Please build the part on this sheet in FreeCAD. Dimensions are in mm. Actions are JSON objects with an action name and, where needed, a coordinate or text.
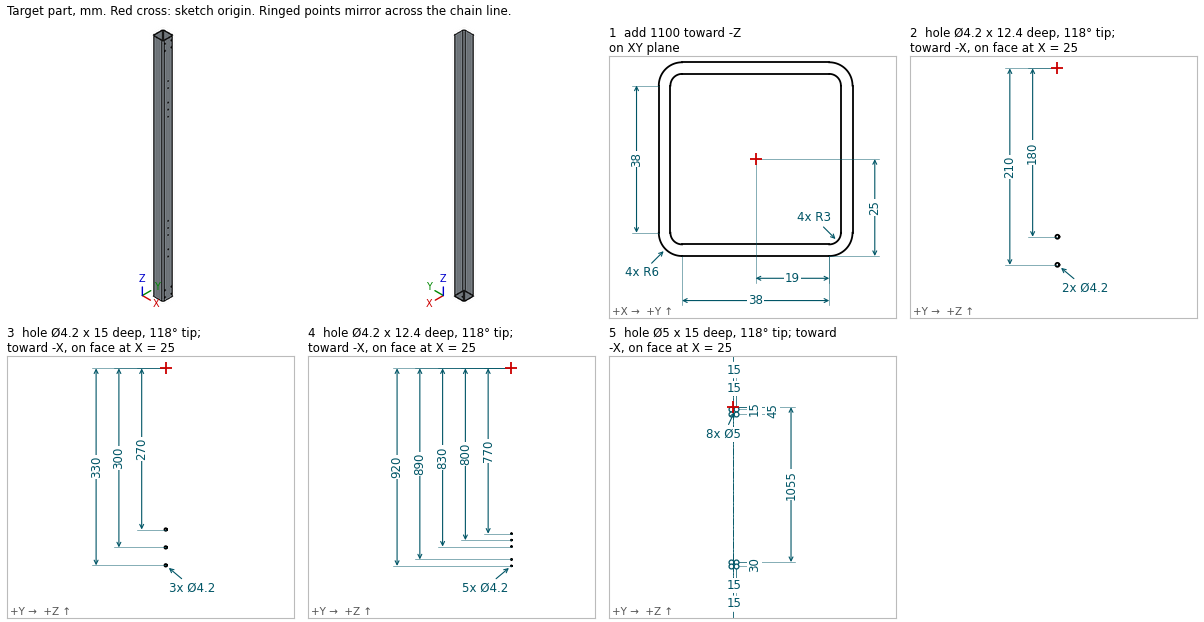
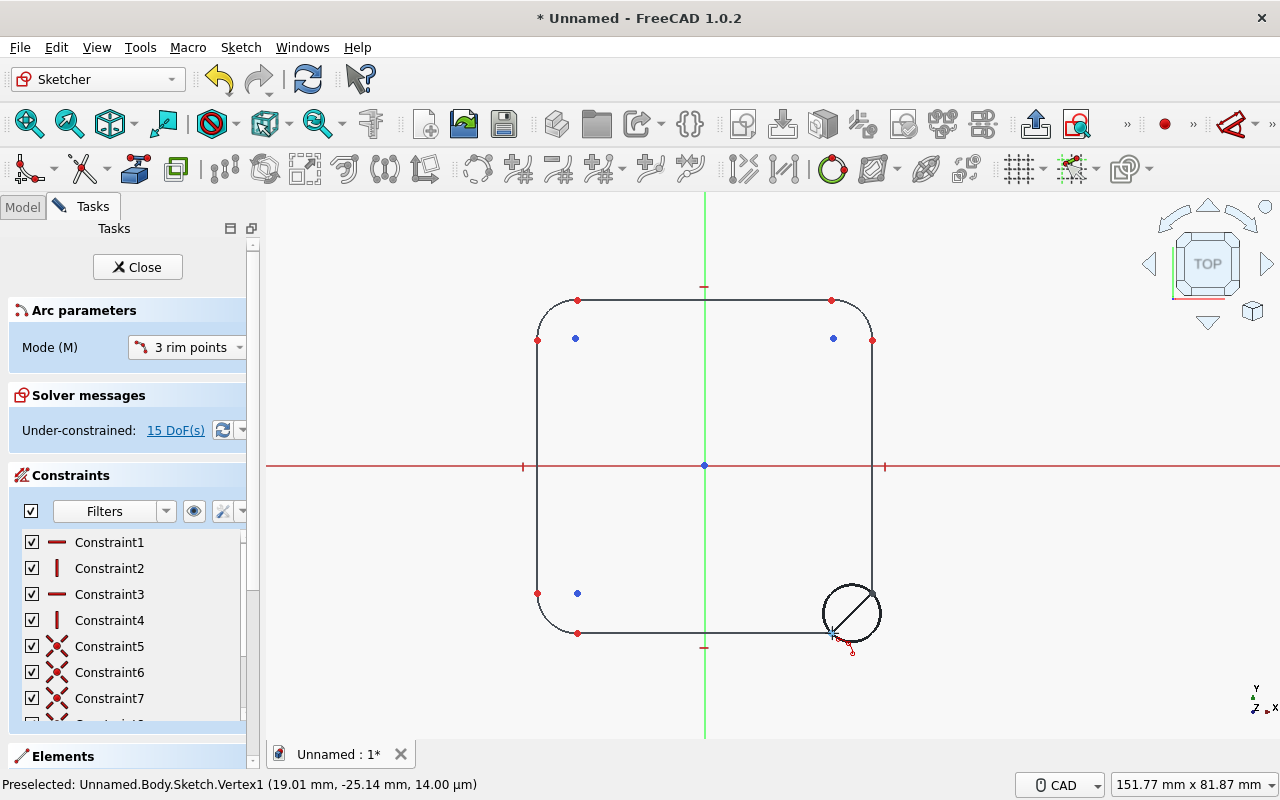
{"action": "scroll", "coordinate": [860, 621], "scroll_direction": "up", "scroll_amount": 2}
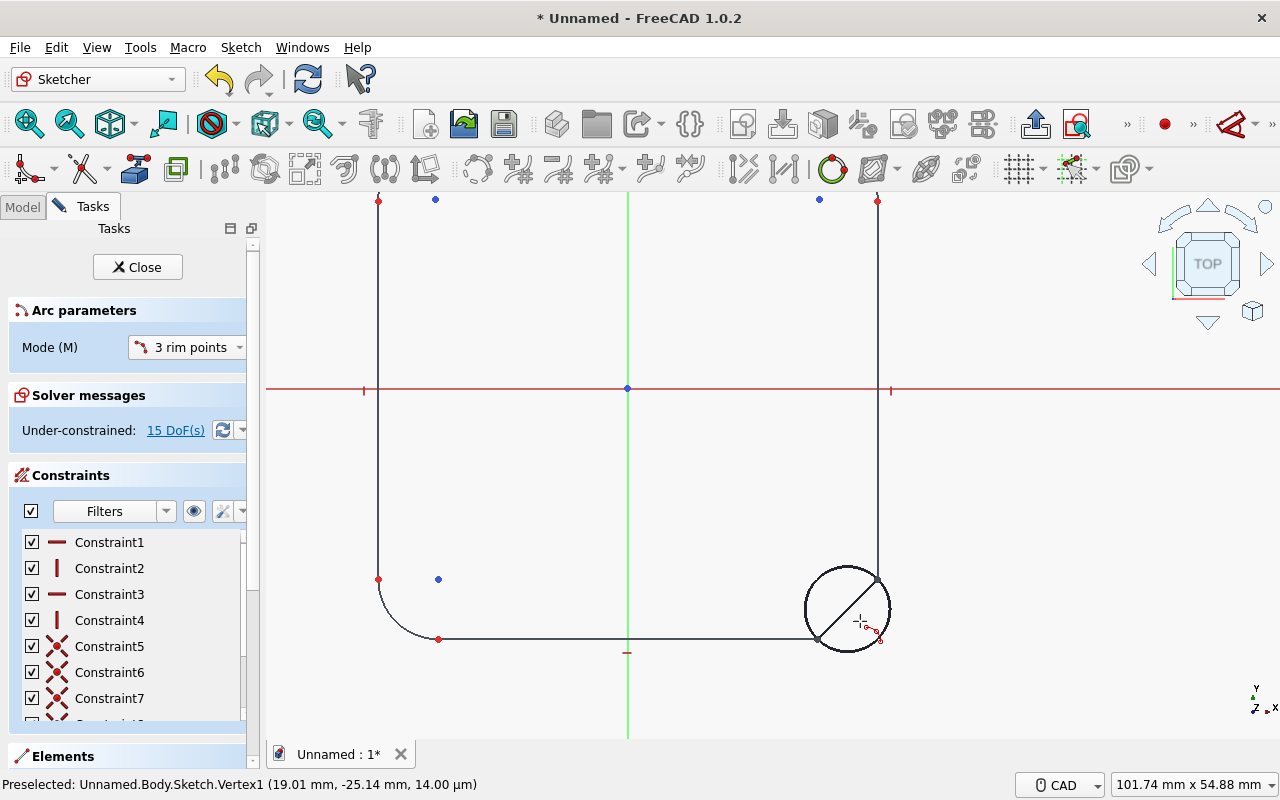
{"action": "left_click", "coordinate": [860, 620]}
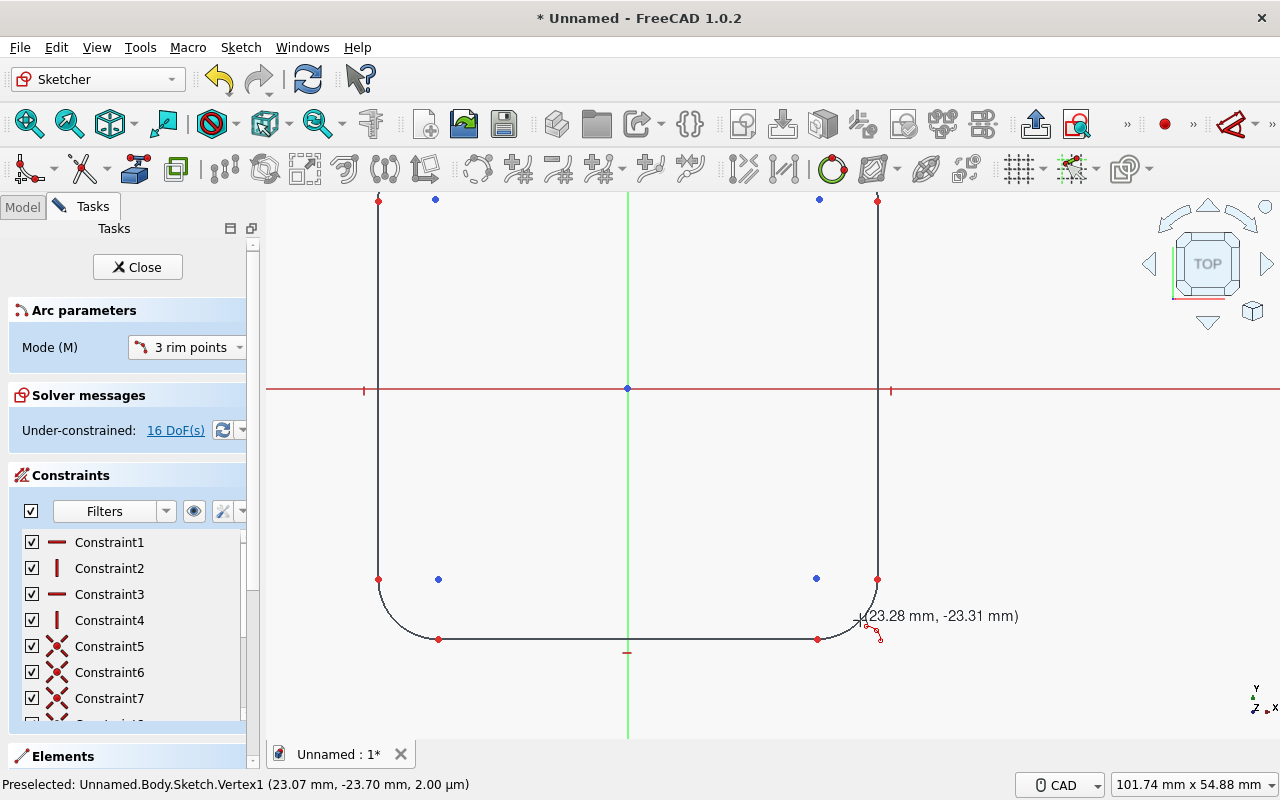
{"action": "key", "text": "g l"}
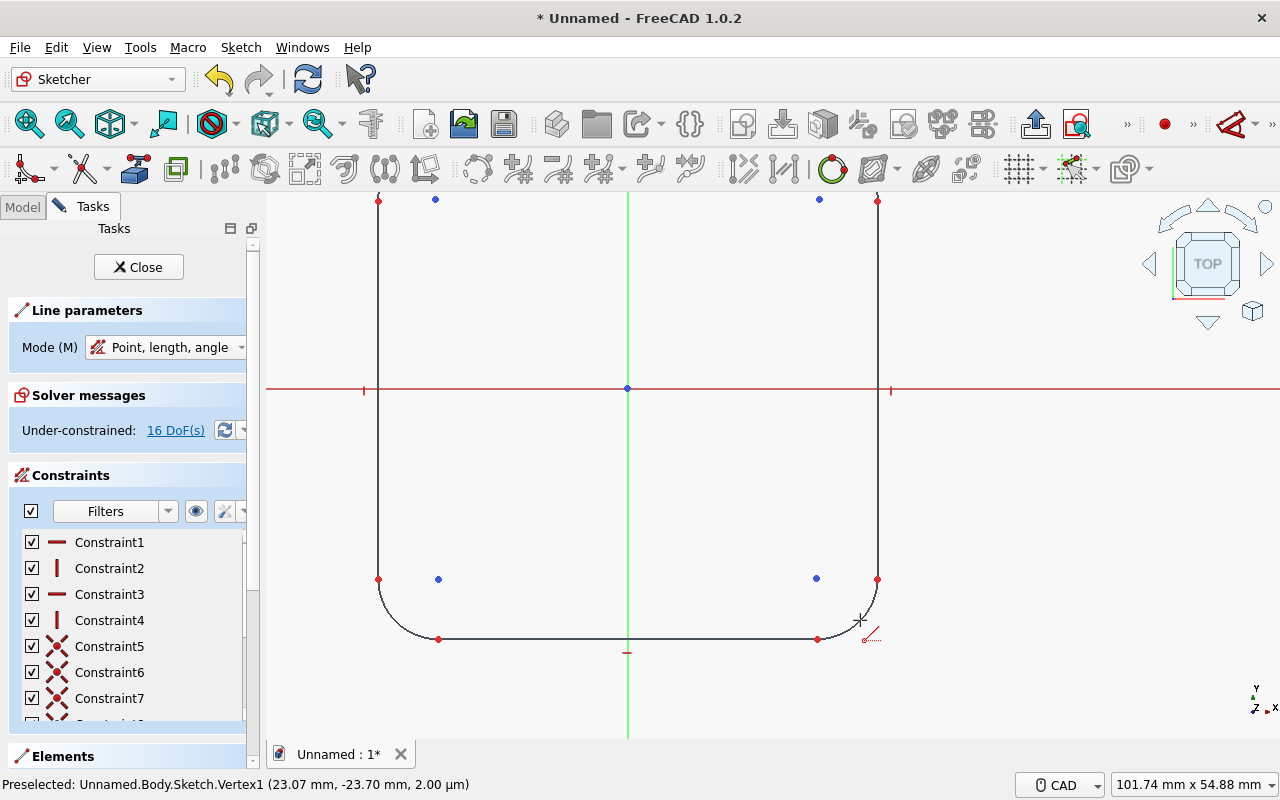
{"action": "left_click", "coordinate": [439, 608]}
{"action": "left_click", "coordinate": [817, 608]}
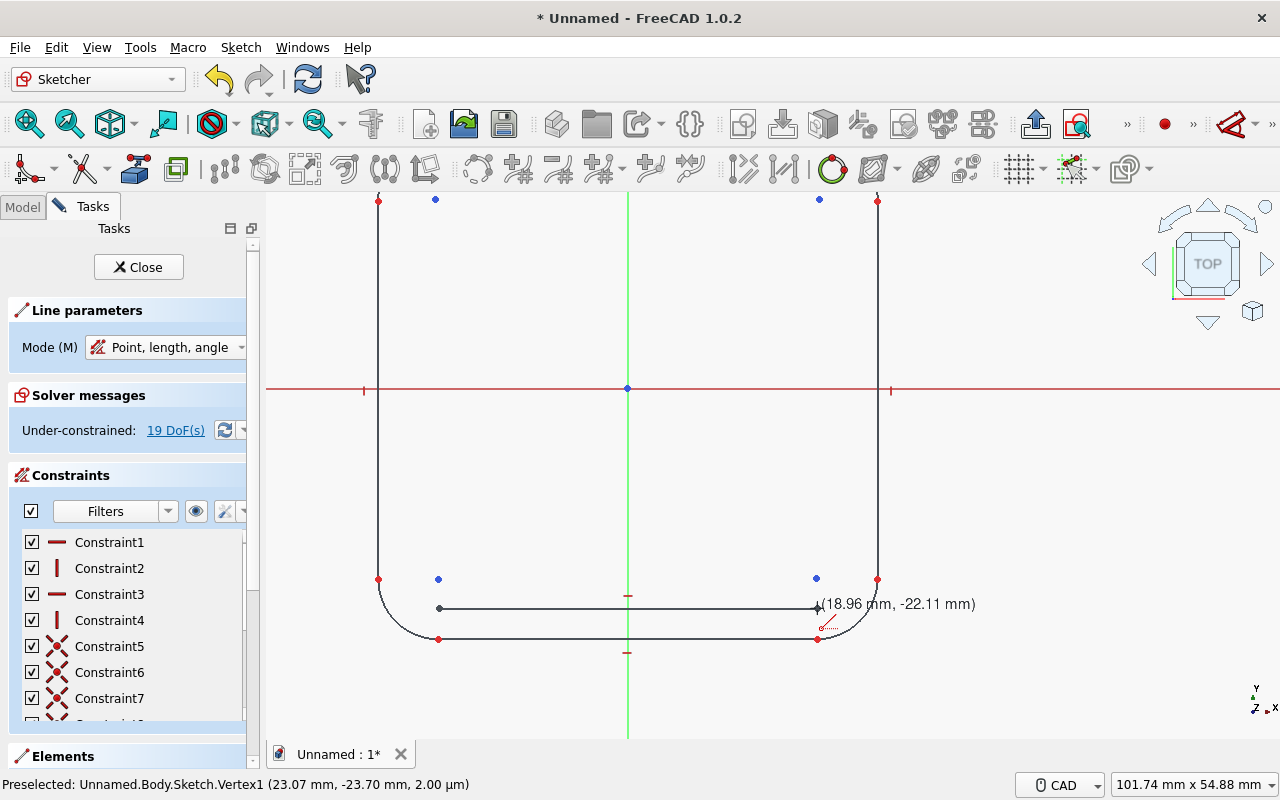
{"action": "left_click", "coordinate": [847, 578]}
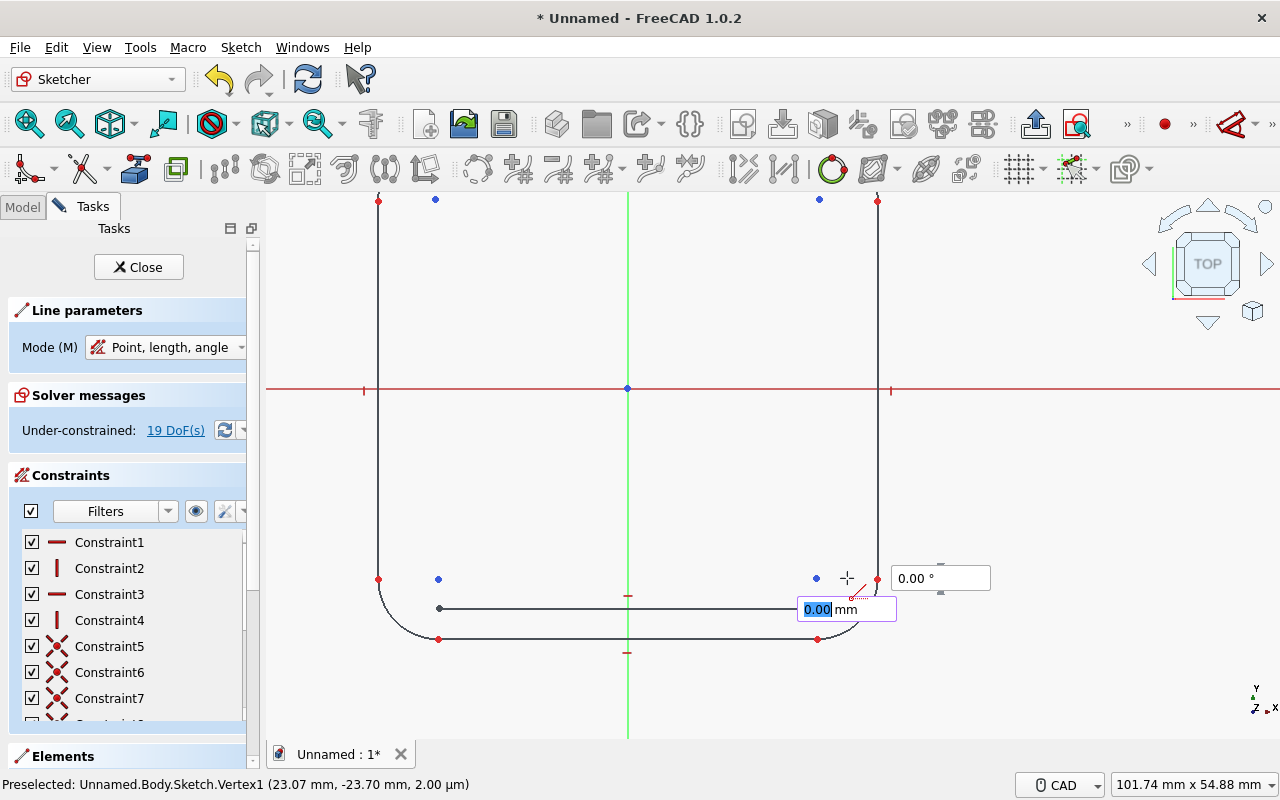
{"action": "scroll", "coordinate": [860, 622], "scroll_direction": "down", "scroll_amount": 2}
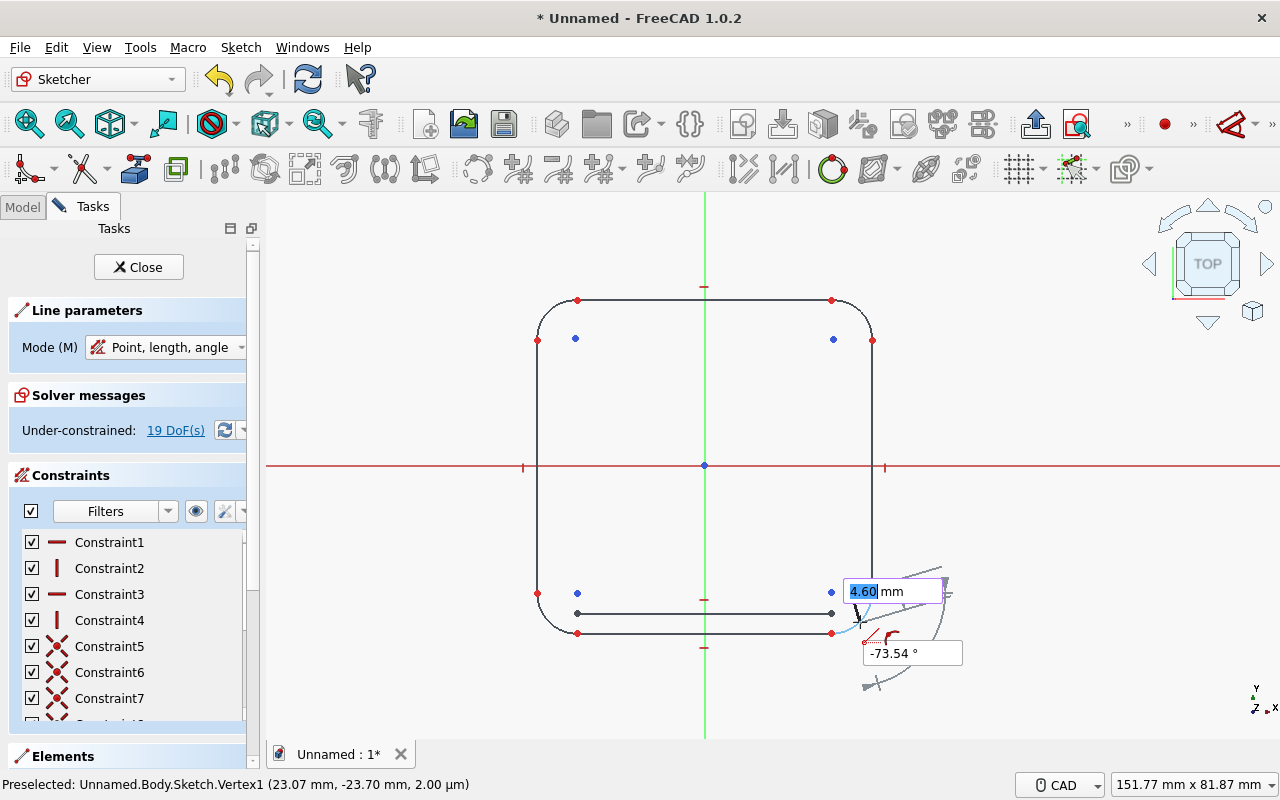
{"action": "left_click", "coordinate": [851, 339]}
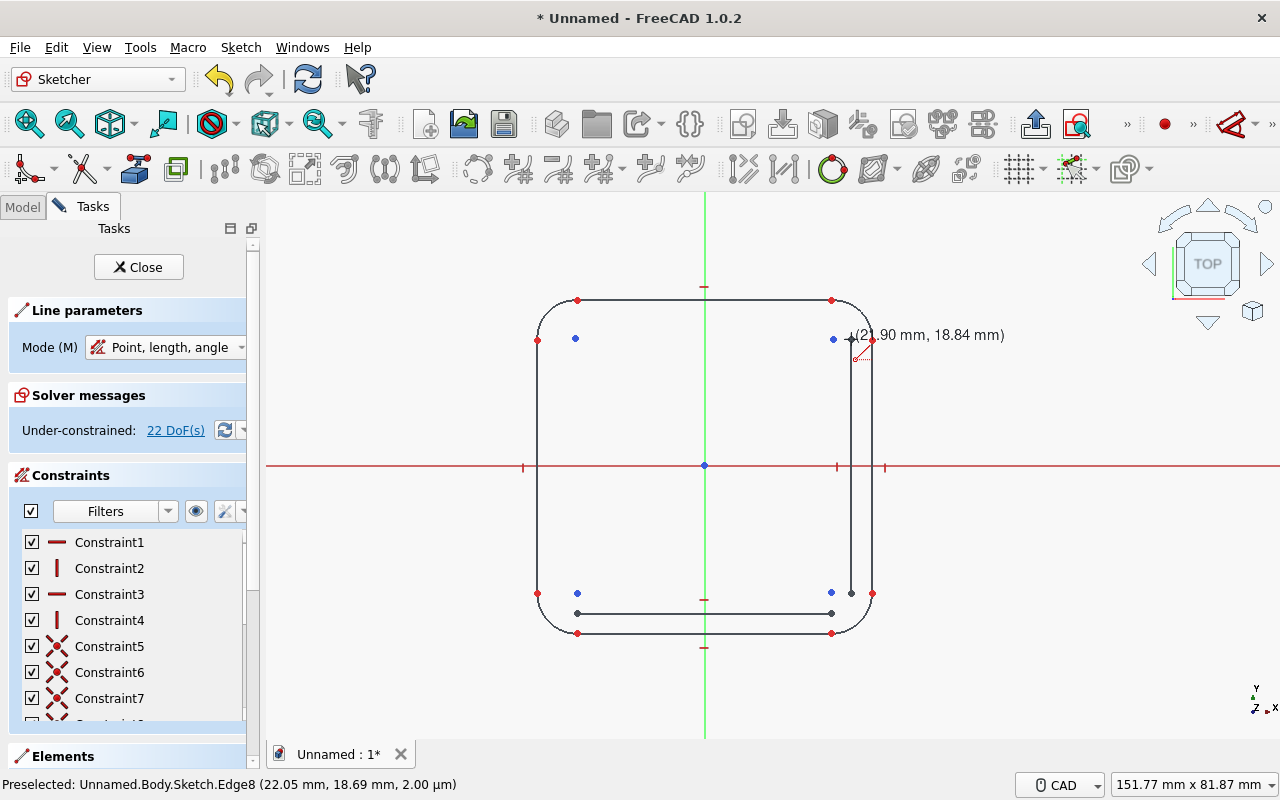
{"action": "left_click", "coordinate": [832, 319]}
{"action": "left_click", "coordinate": [578, 319]}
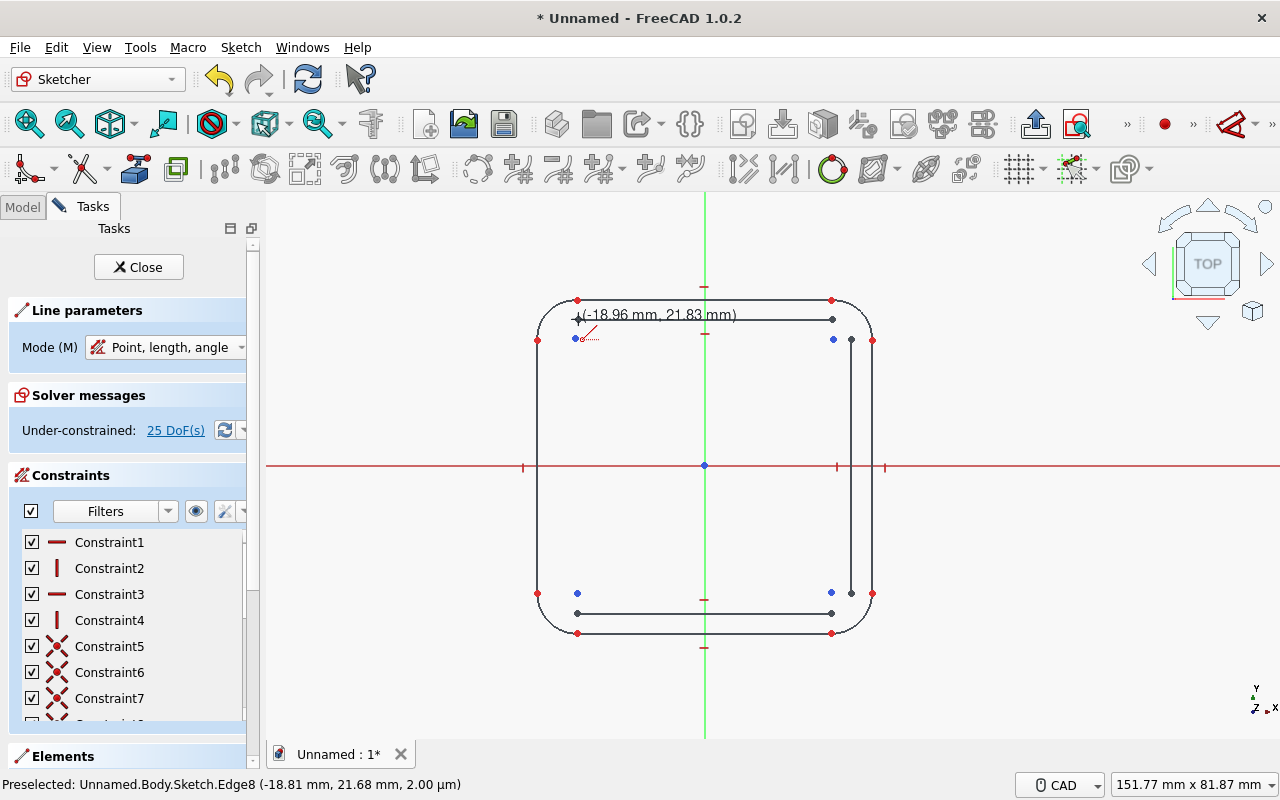
{"action": "left_click", "coordinate": [558, 339]}
{"action": "left_click", "coordinate": [558, 593]}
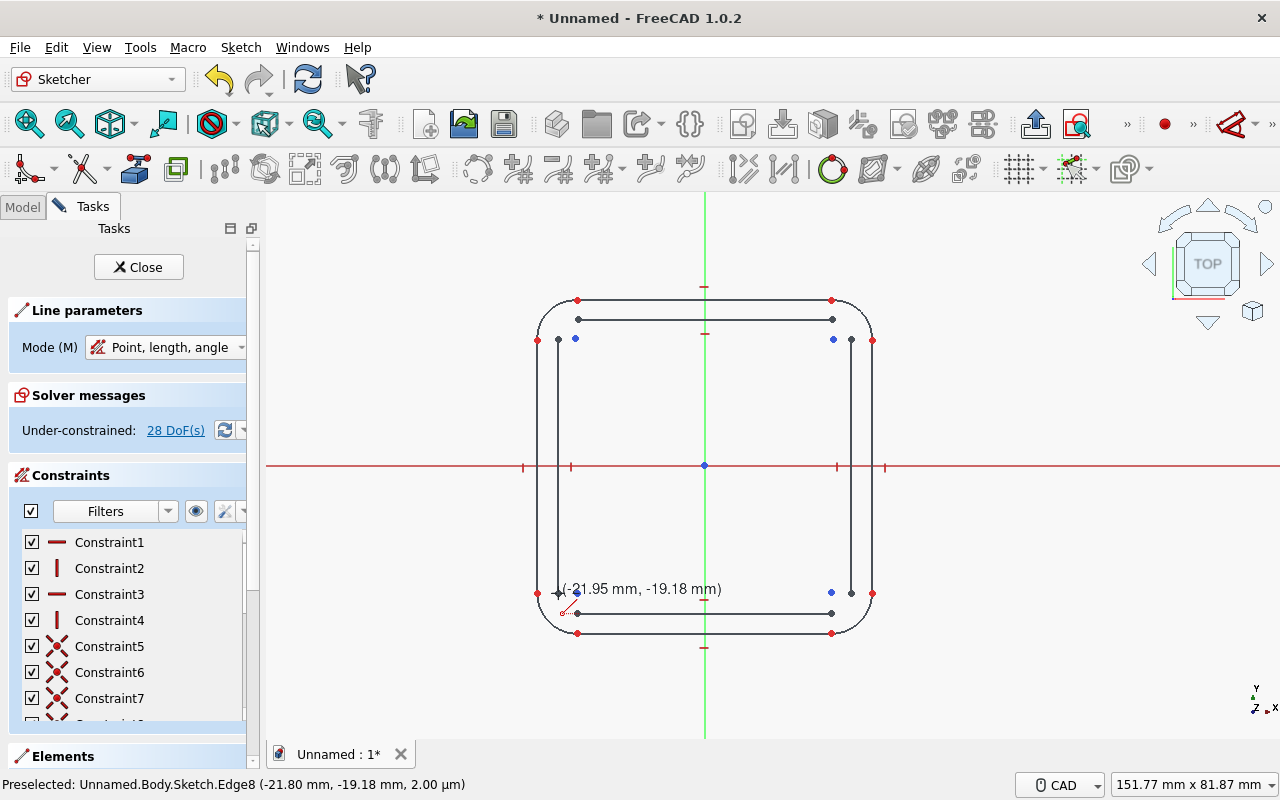
{"action": "key", "text": "g 3 a"}